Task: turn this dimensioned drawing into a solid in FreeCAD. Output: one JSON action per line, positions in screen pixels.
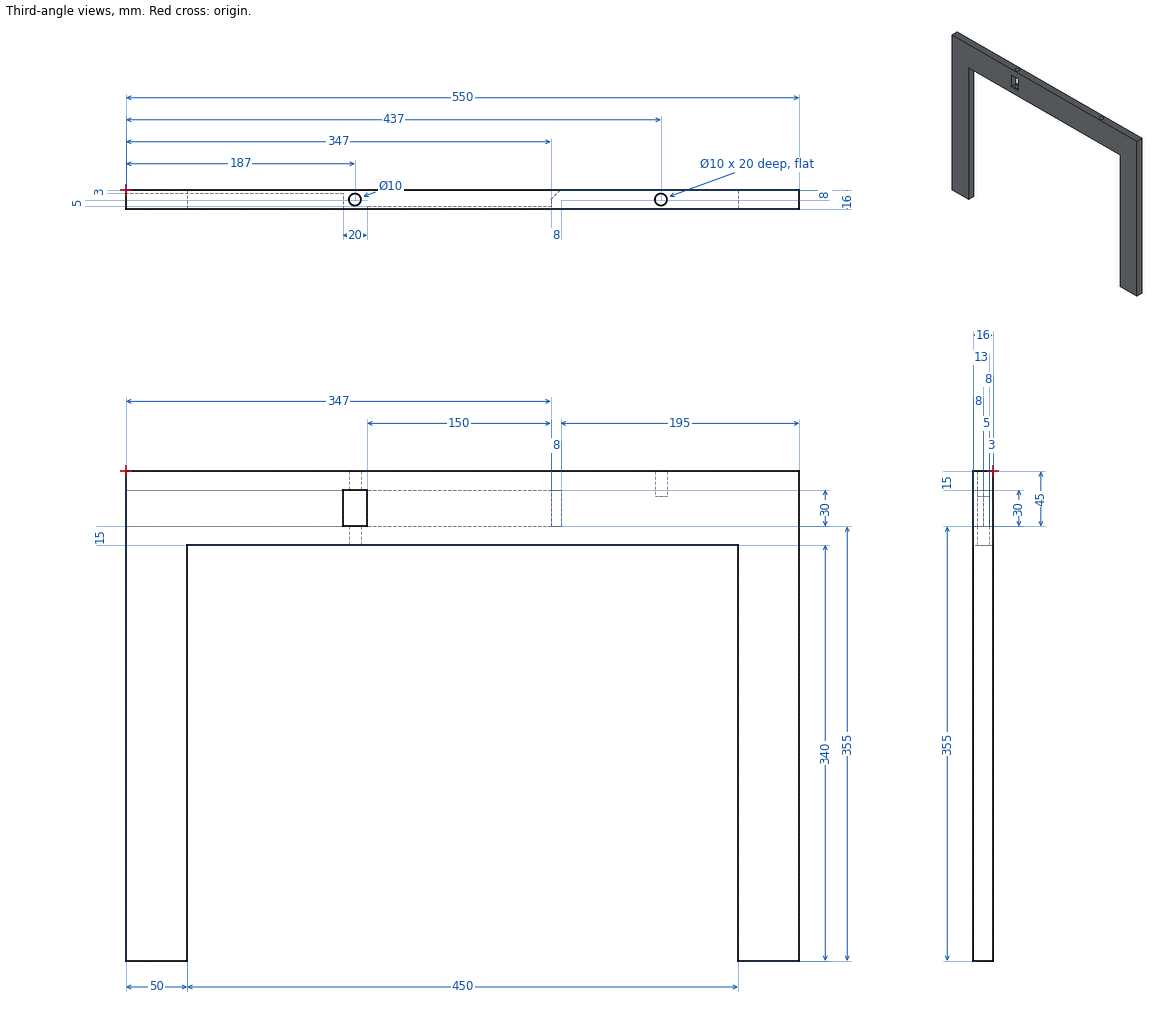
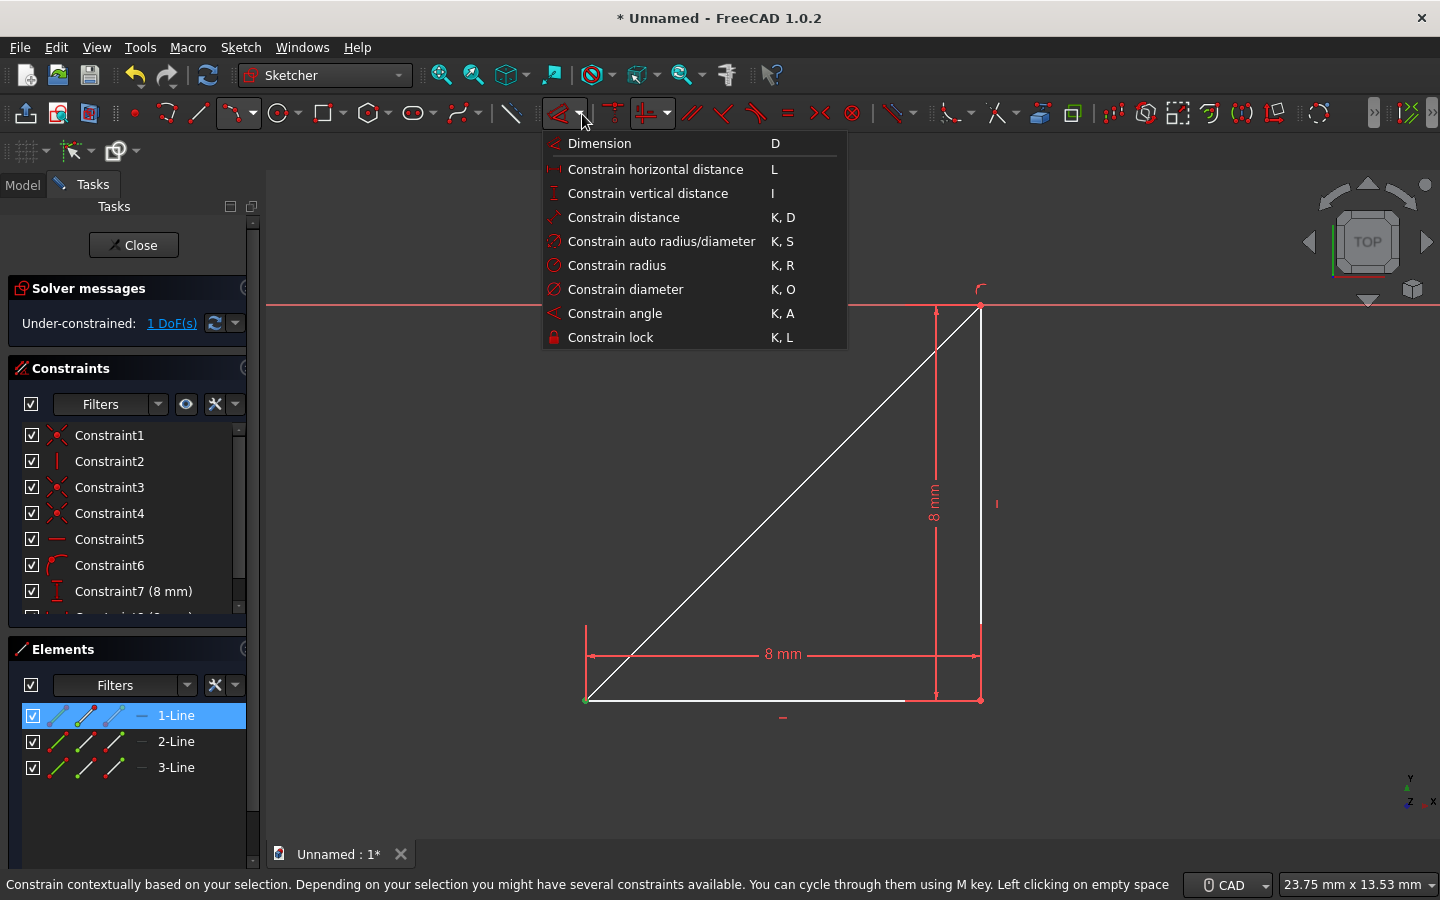
{"action": "left_click", "coordinate": [695, 169]}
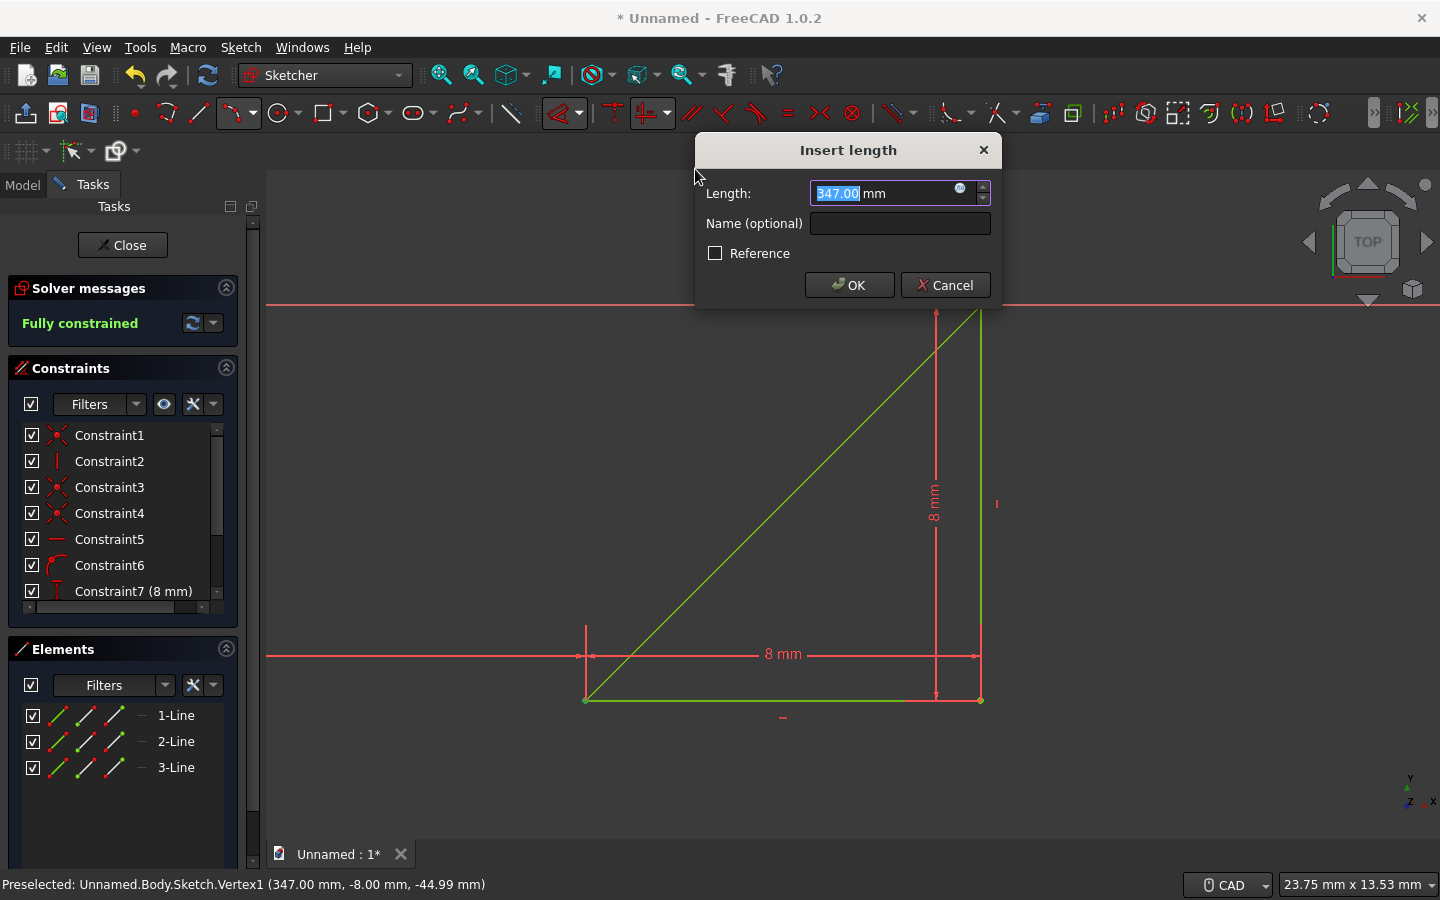
{"action": "type", "text": "347"}
{"action": "key", "text": "Return"}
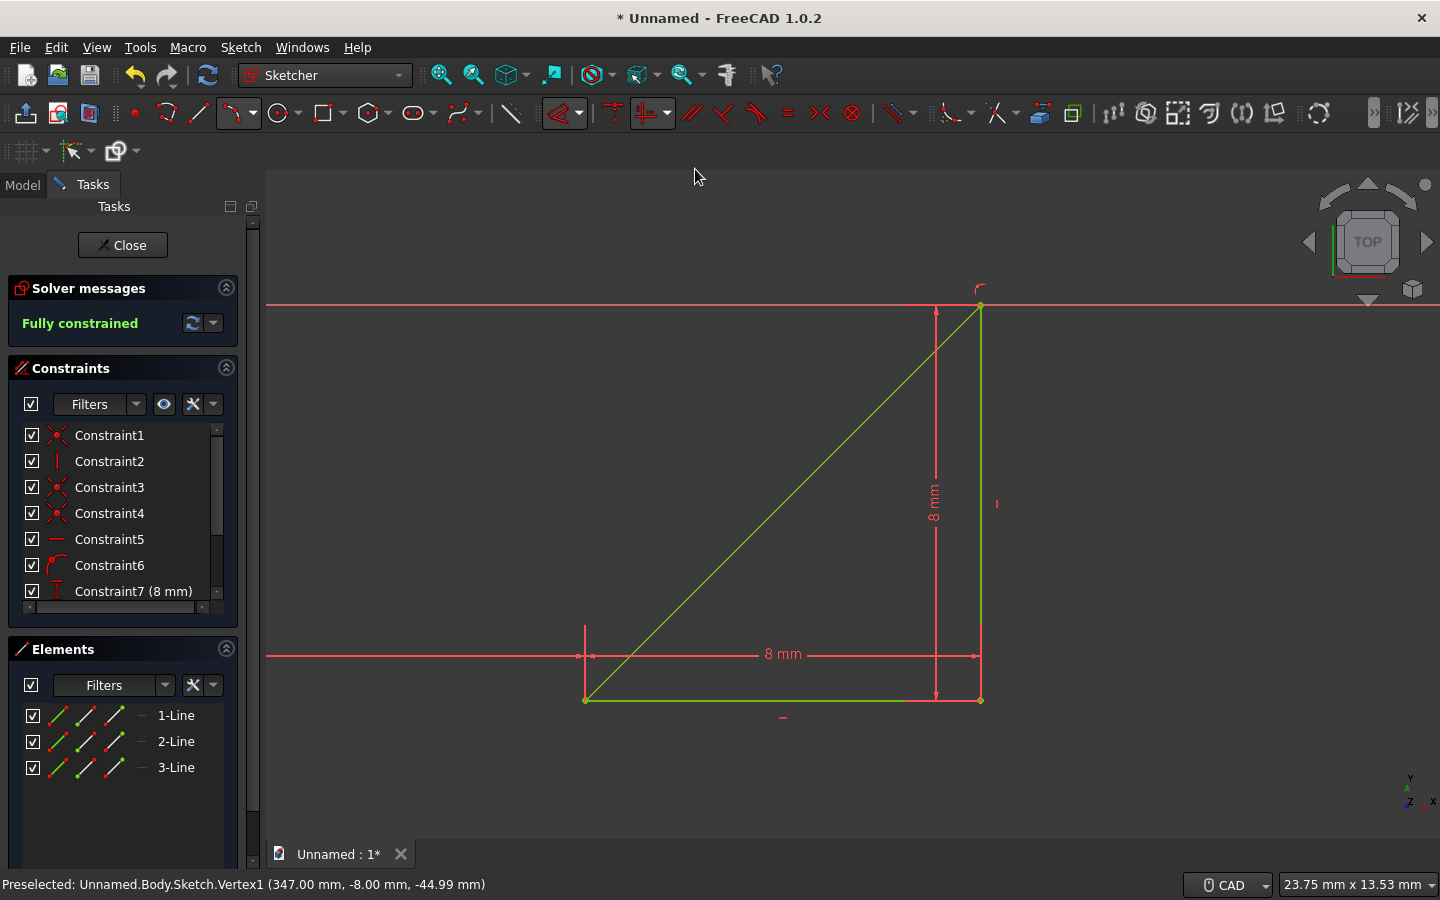
{"action": "left_click", "coordinate": [123, 245]}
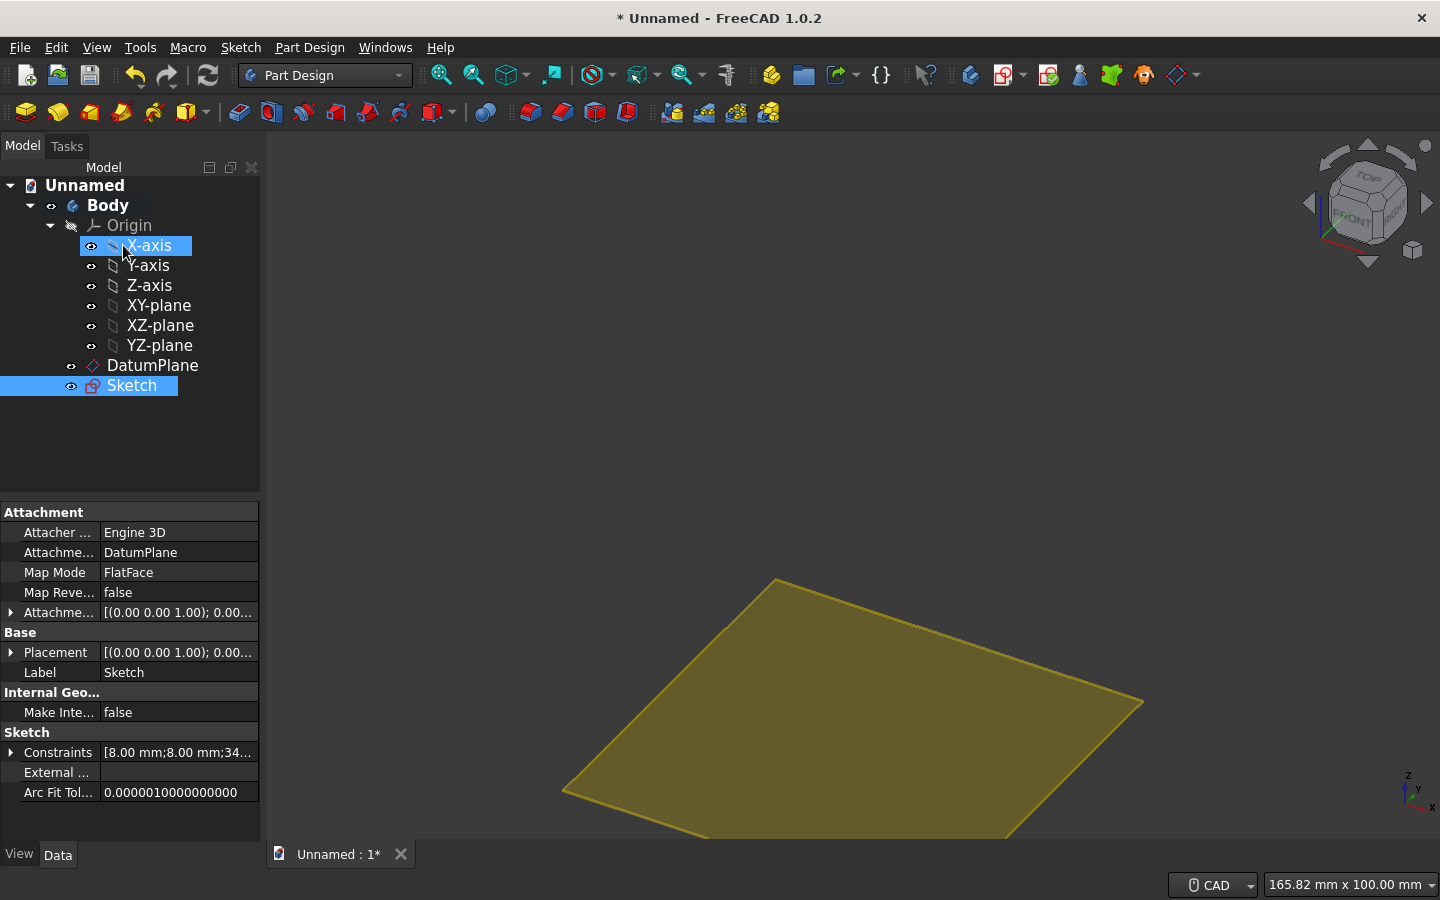
{"action": "left_click", "coordinate": [26, 112]}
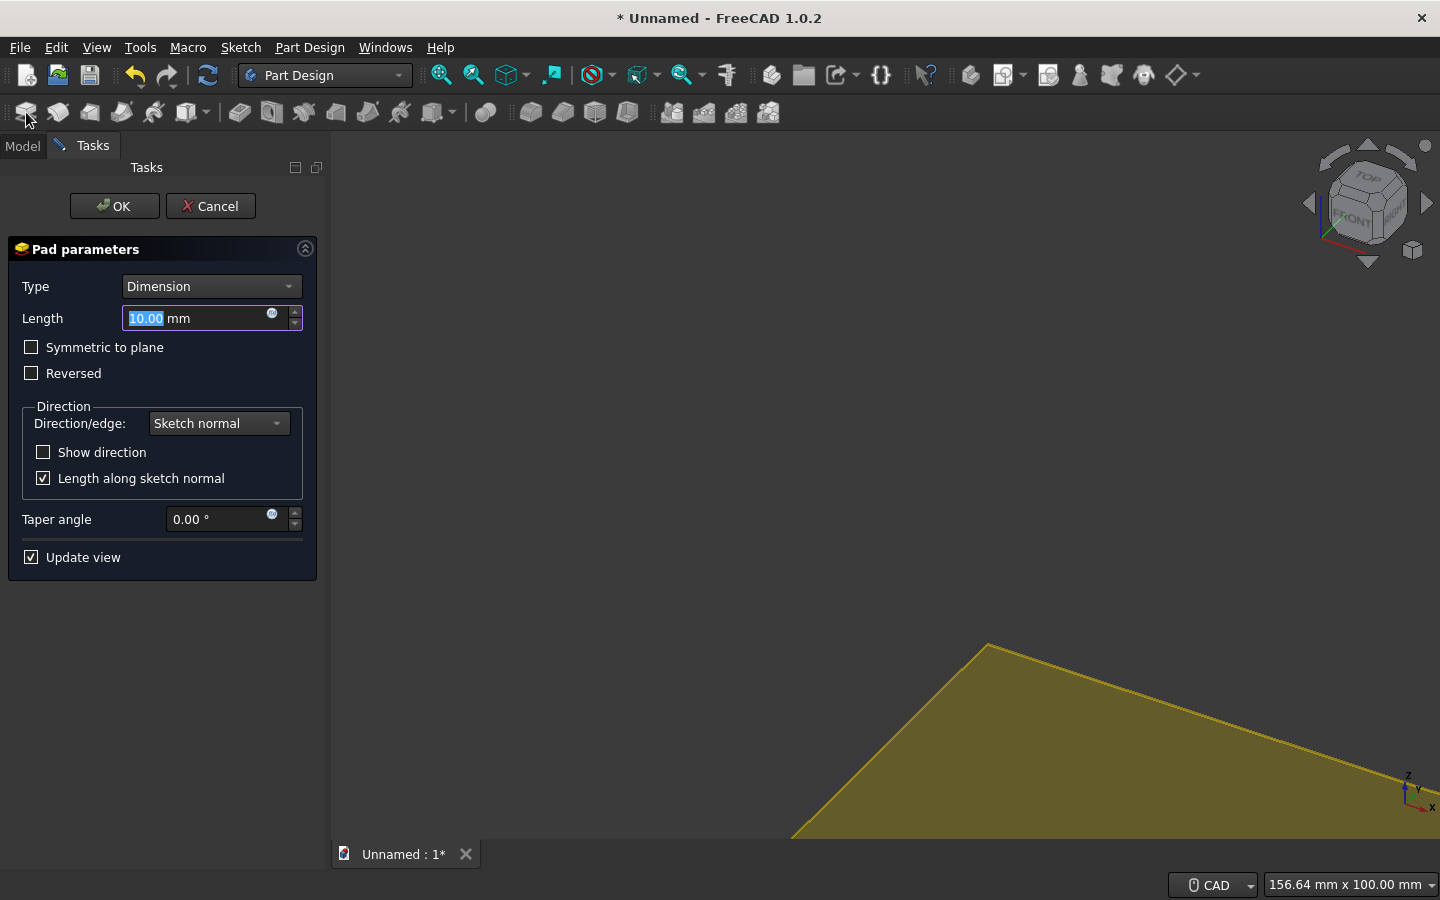
{"action": "type", "text": "30"}
{"action": "key", "text": "Tab"}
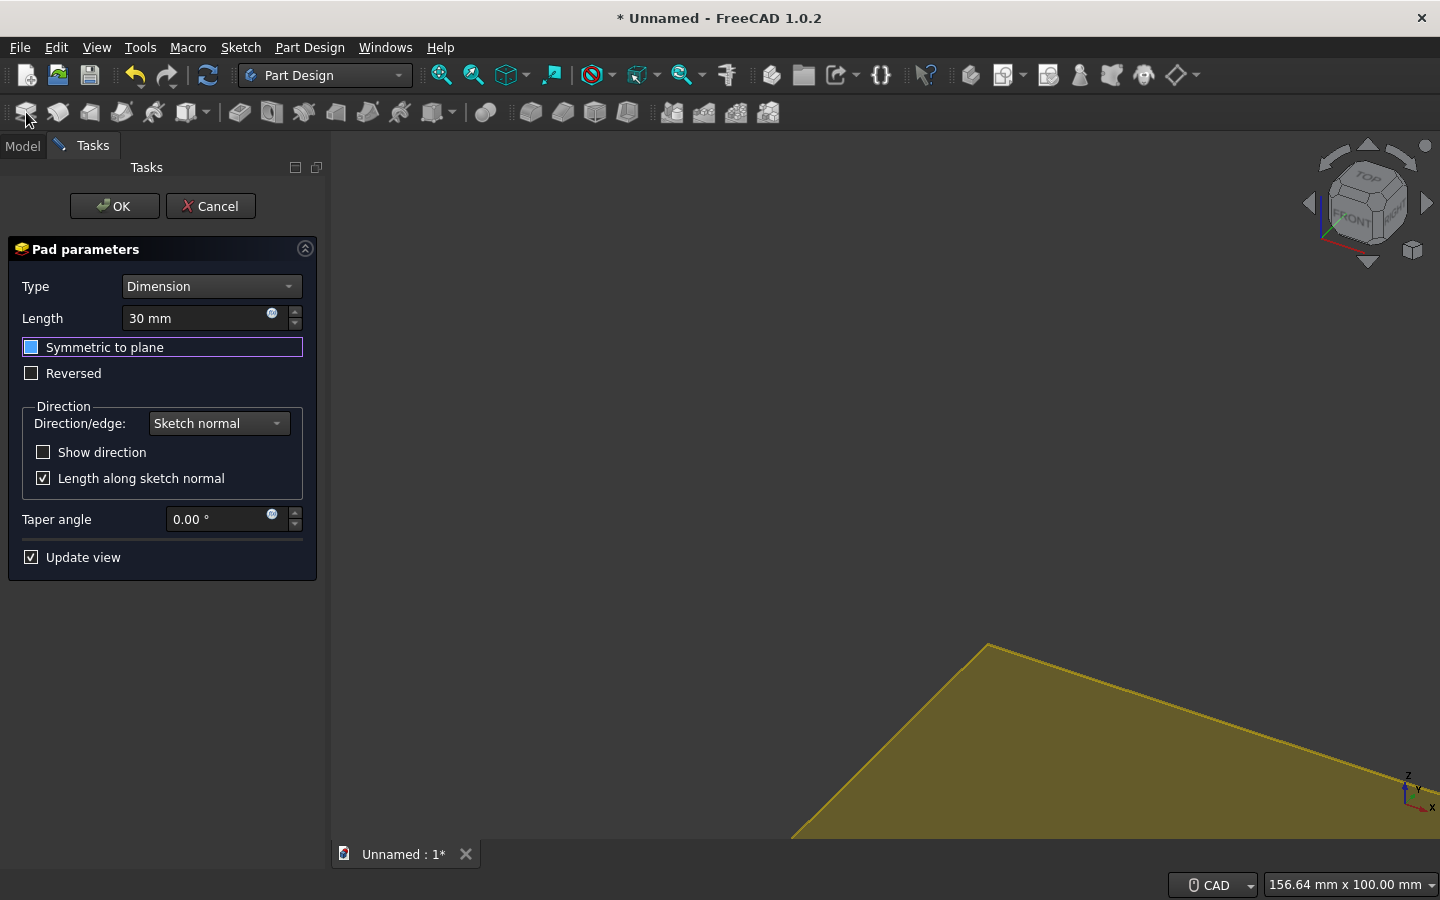
{"action": "left_click", "coordinate": [115, 206]}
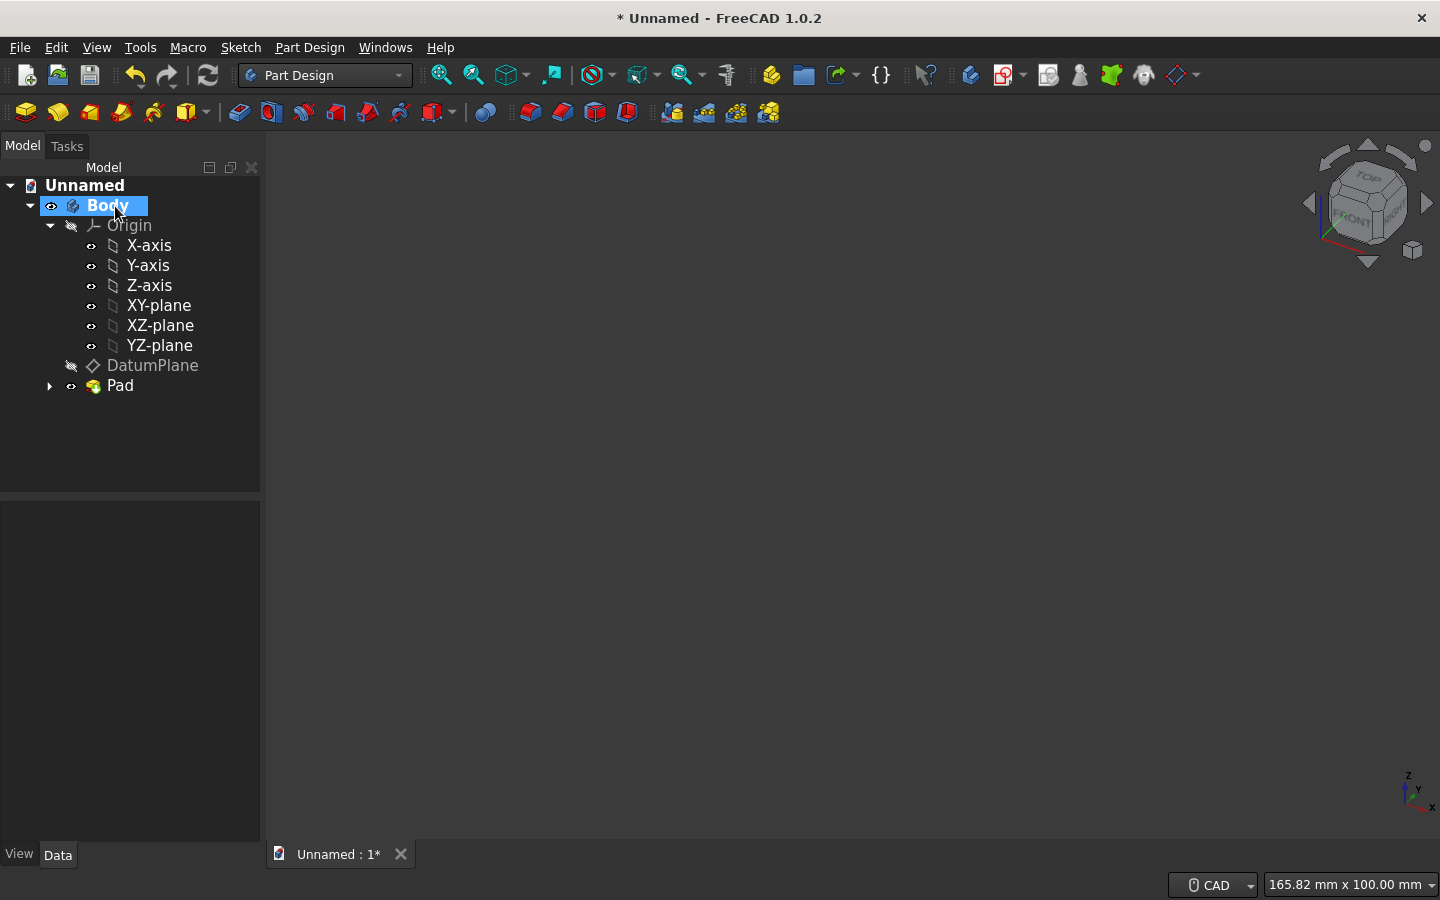
{"action": "left_click", "coordinate": [442, 76]}